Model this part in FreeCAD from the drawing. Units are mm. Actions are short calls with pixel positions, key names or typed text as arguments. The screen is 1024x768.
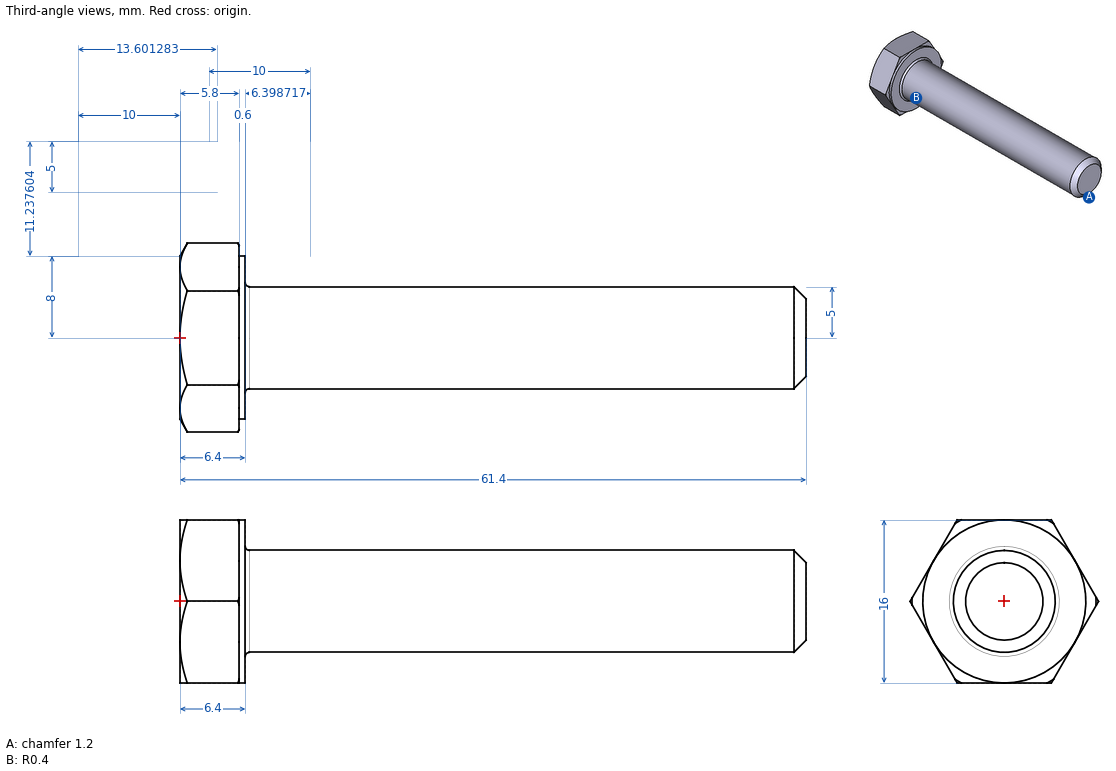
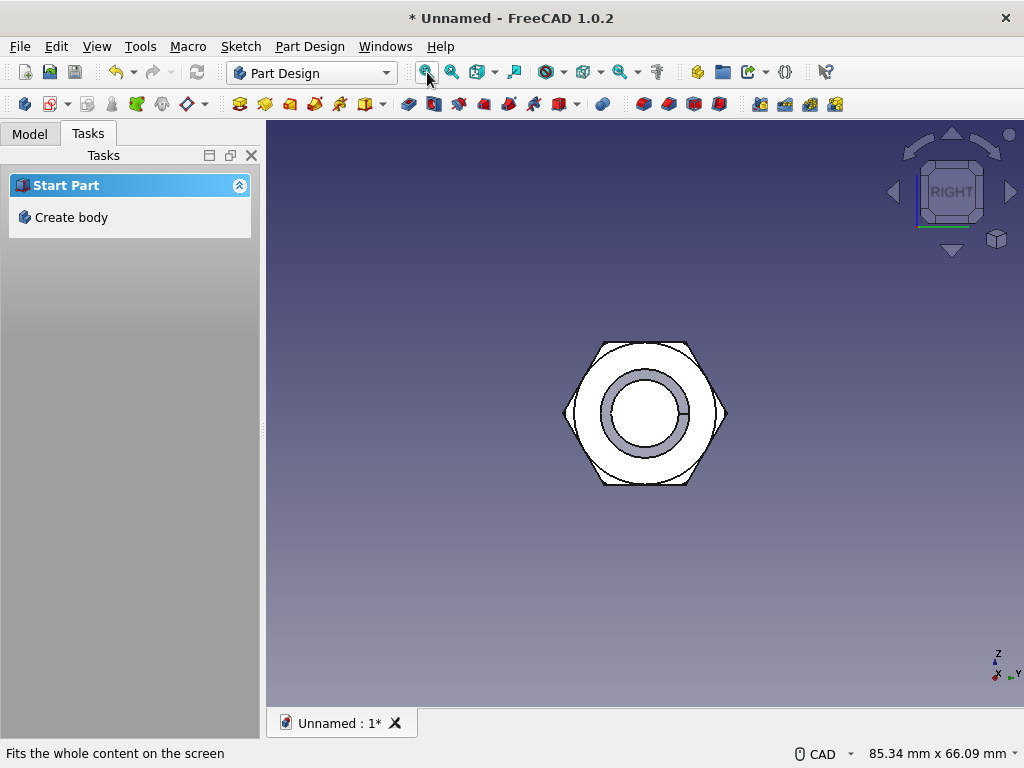
key(5)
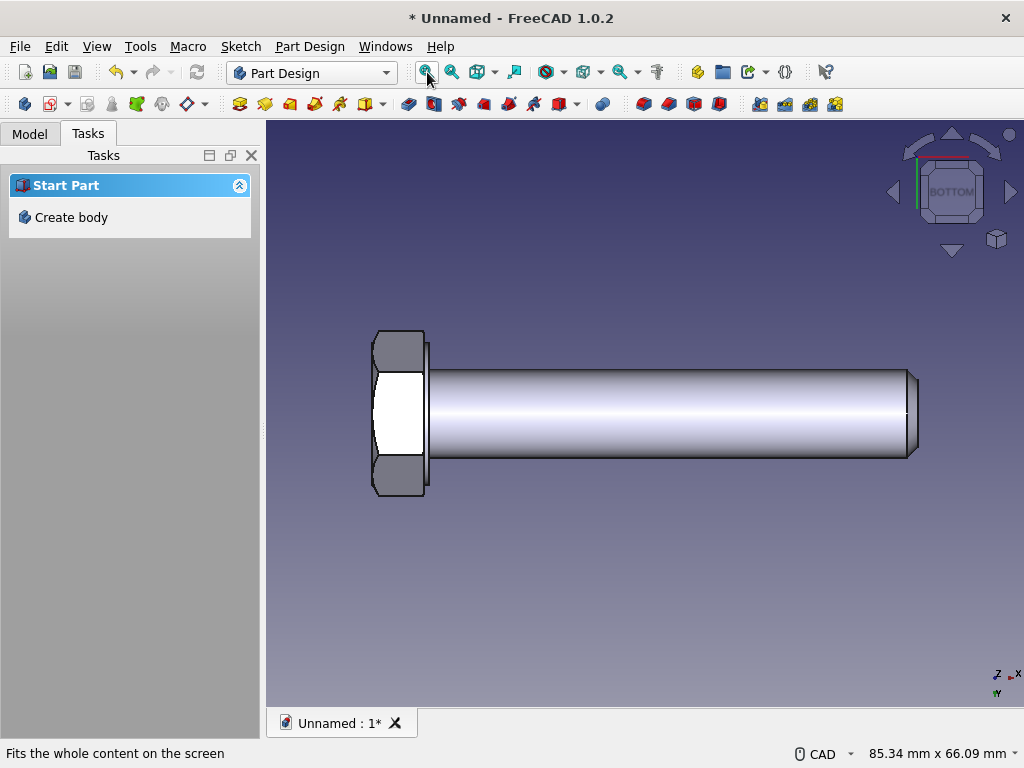
key(4)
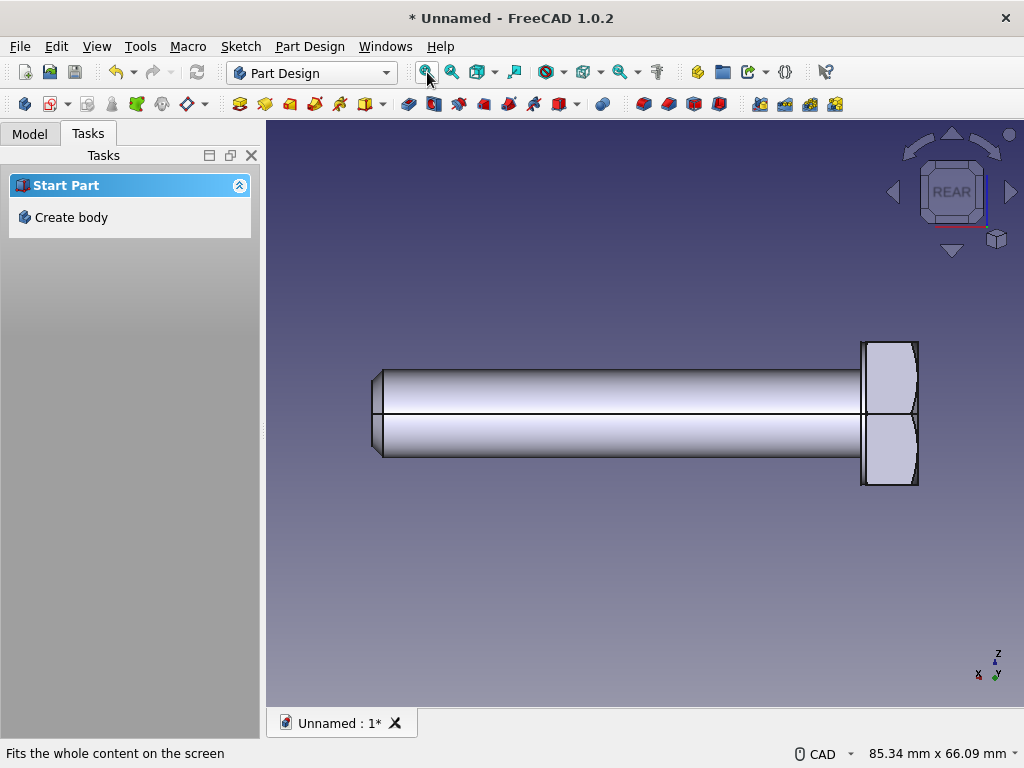
key(6)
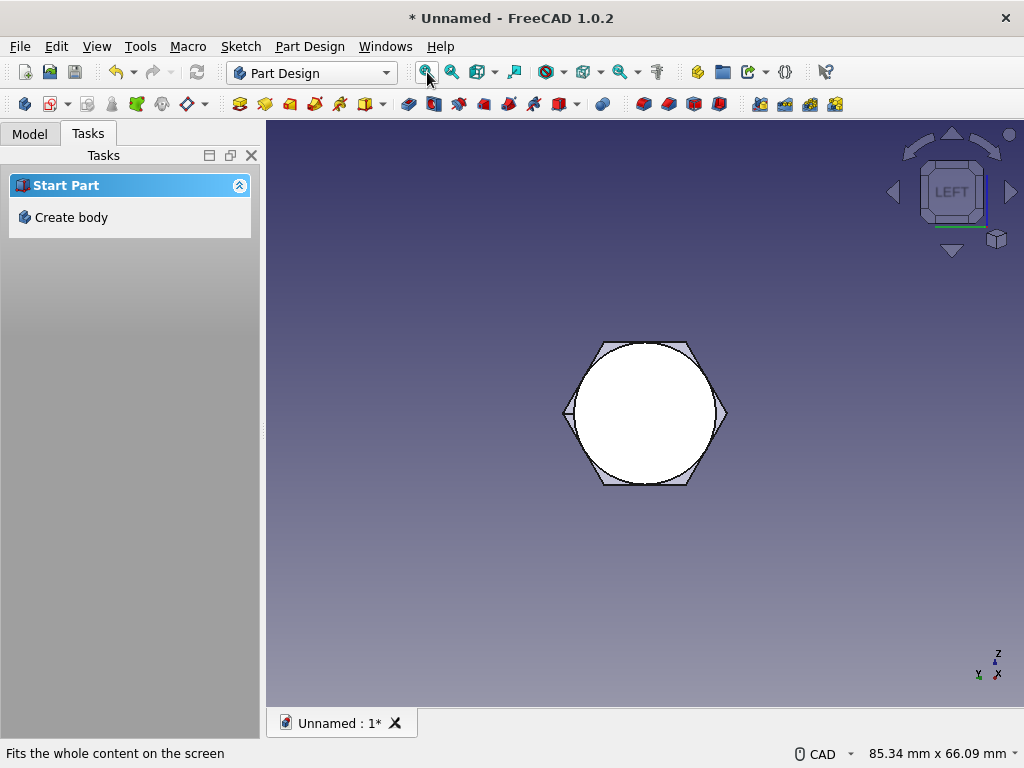
click(427, 72)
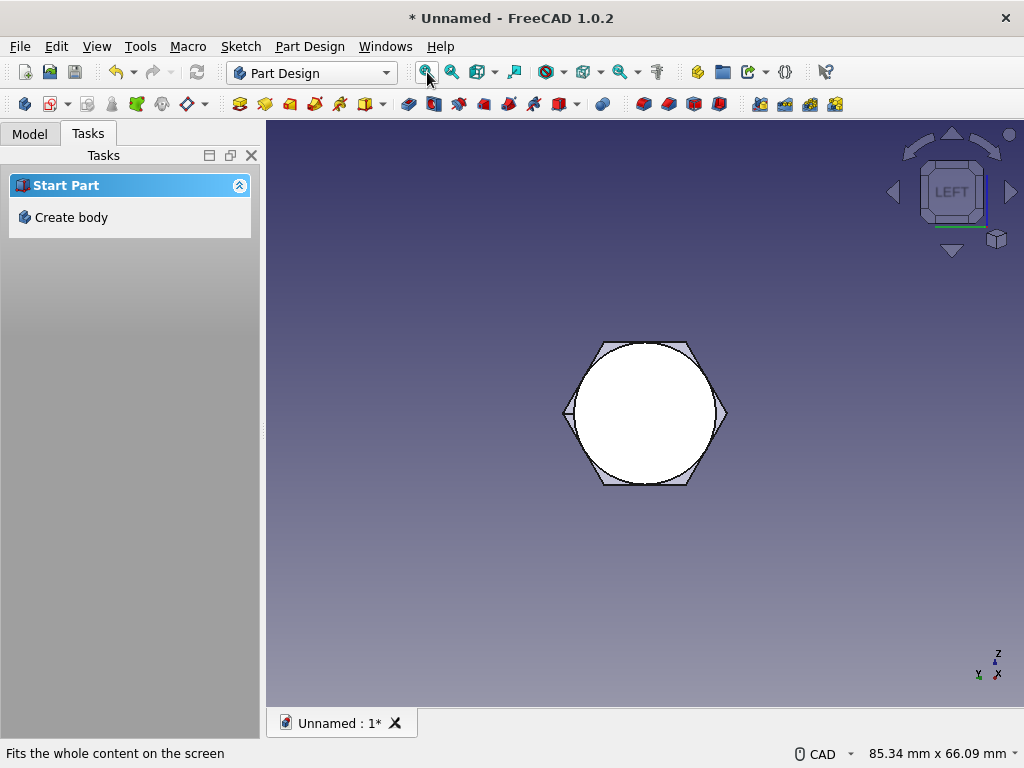
key(v)
key(3)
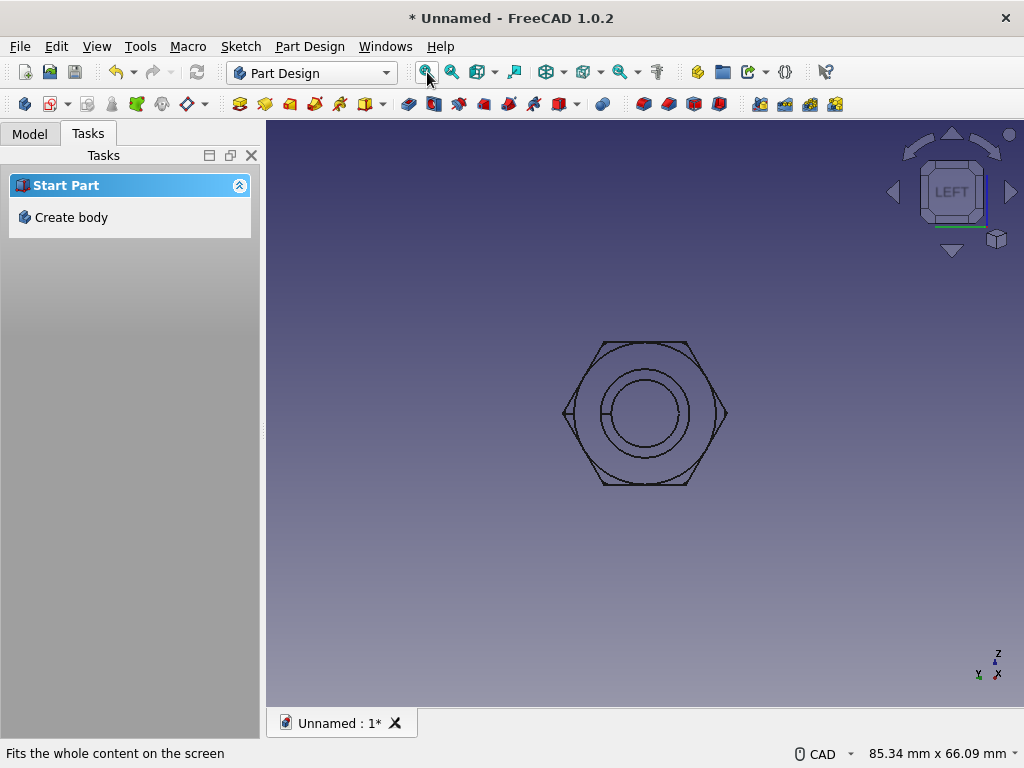
key(0)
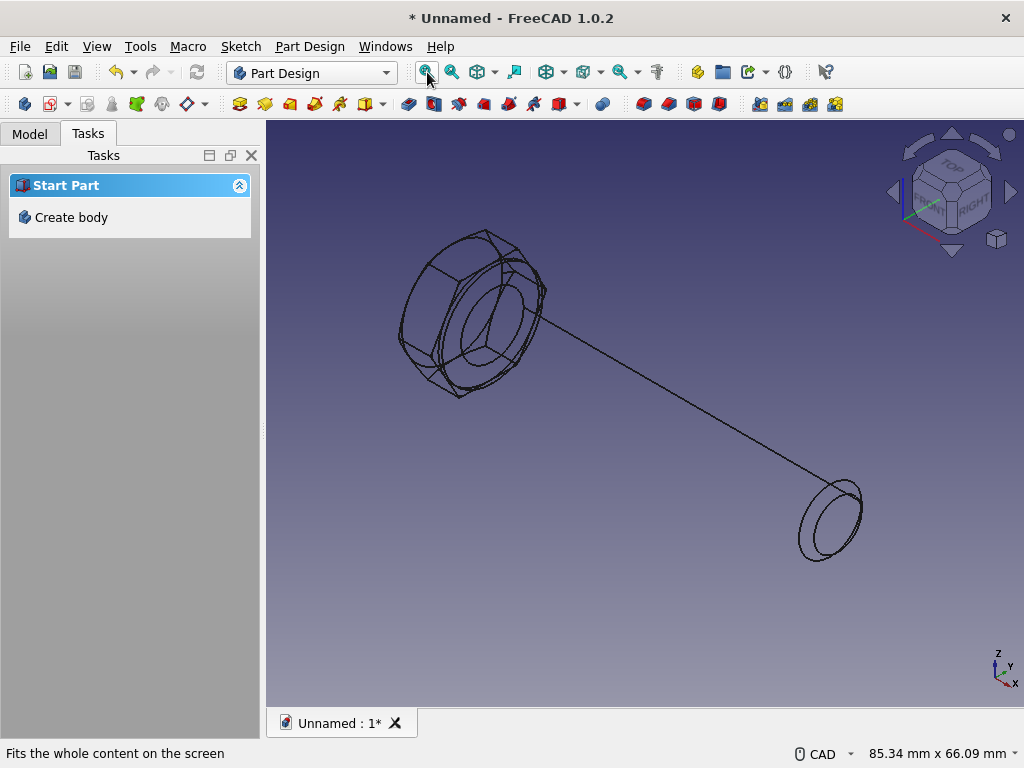
click(461, 343)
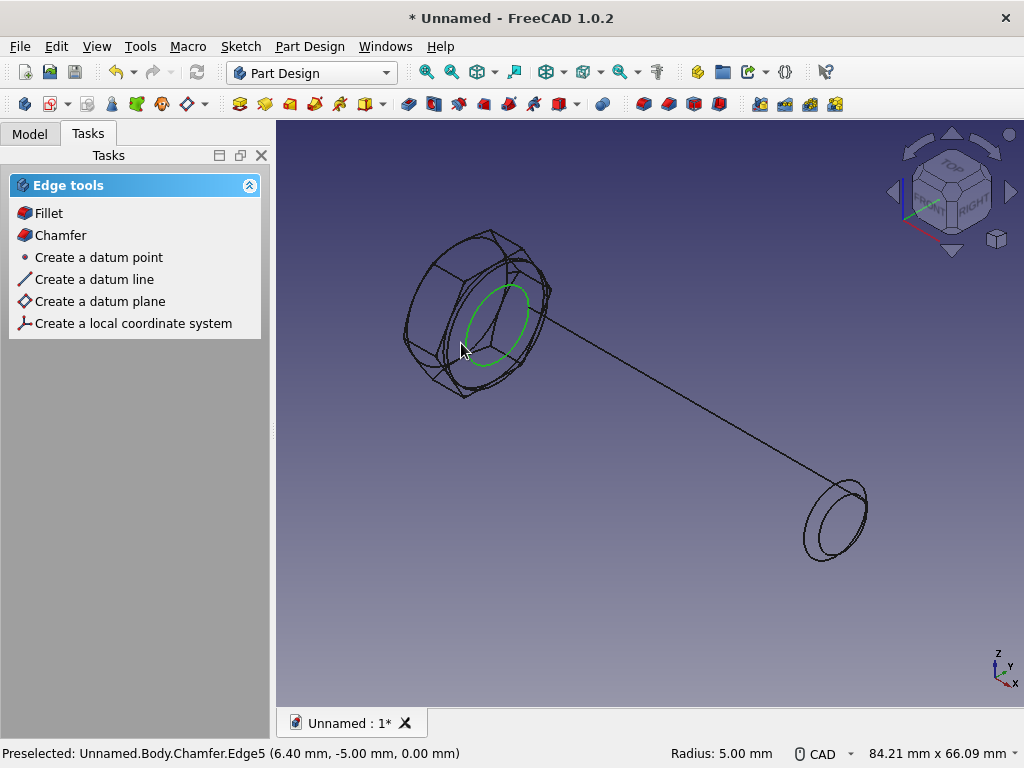
key(v)
key(1)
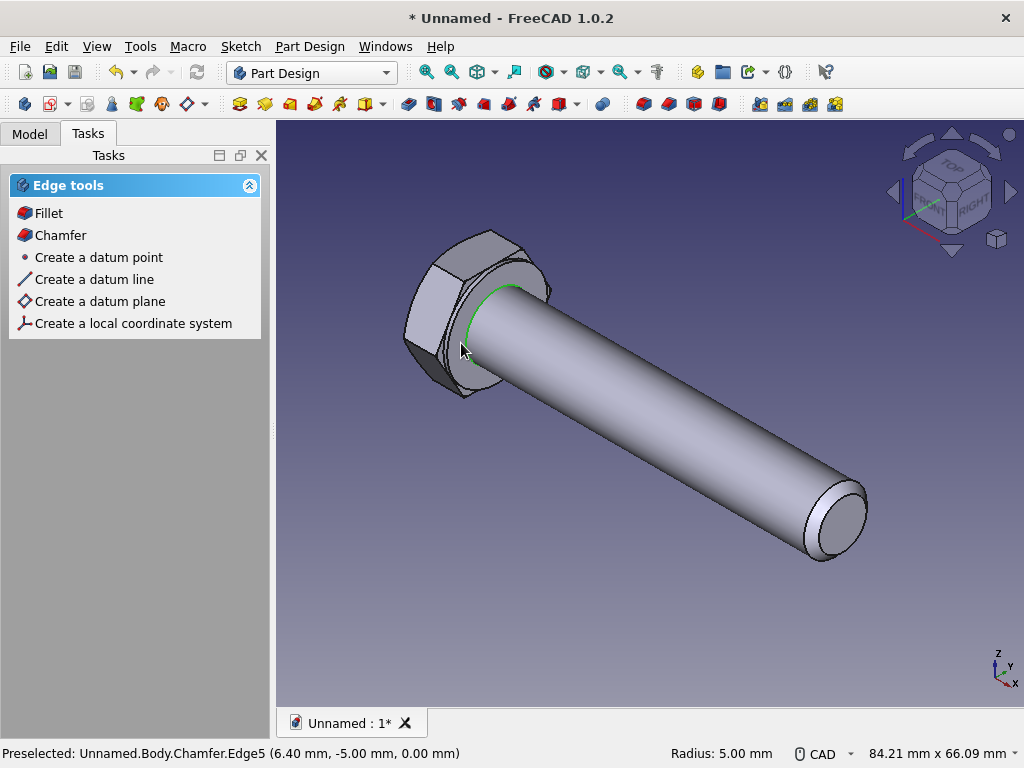
click(644, 104)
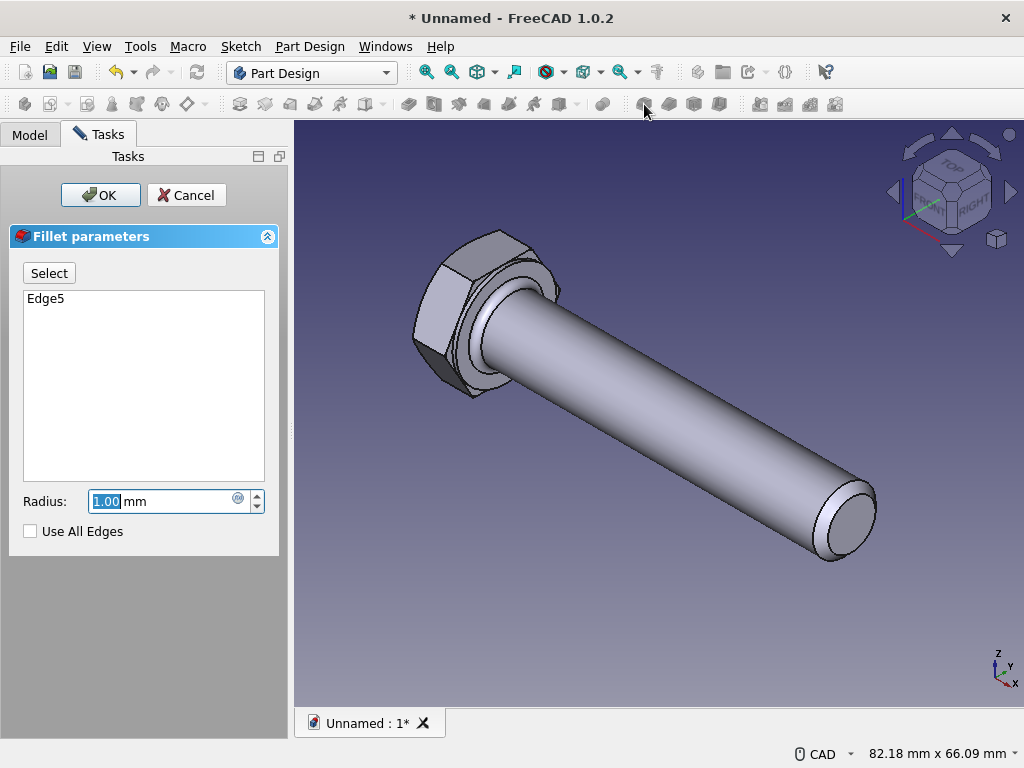
text(0.4)
key(Tab)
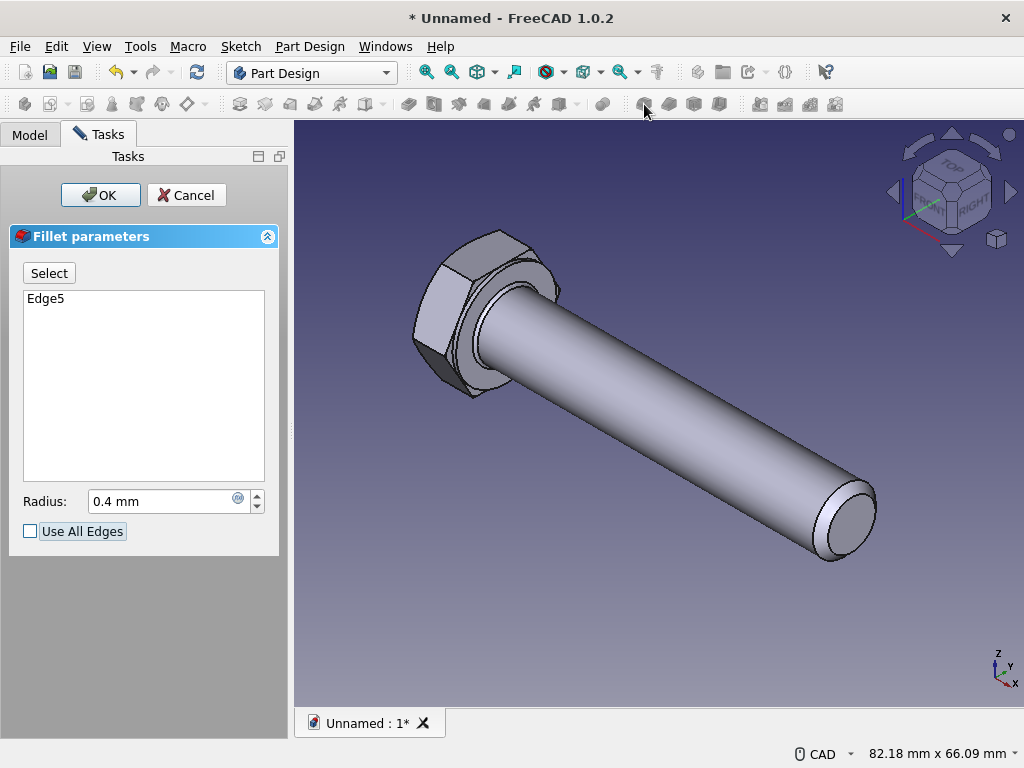
click(101, 195)